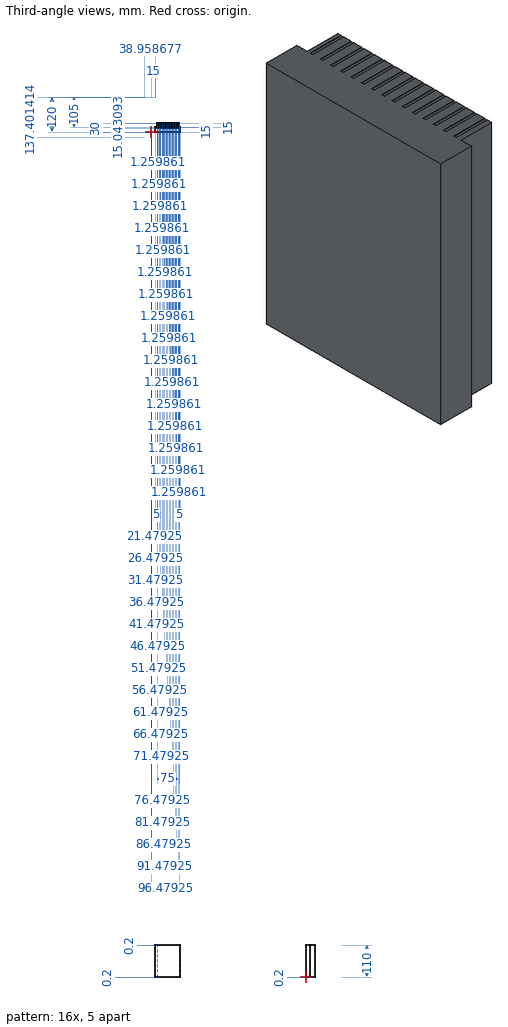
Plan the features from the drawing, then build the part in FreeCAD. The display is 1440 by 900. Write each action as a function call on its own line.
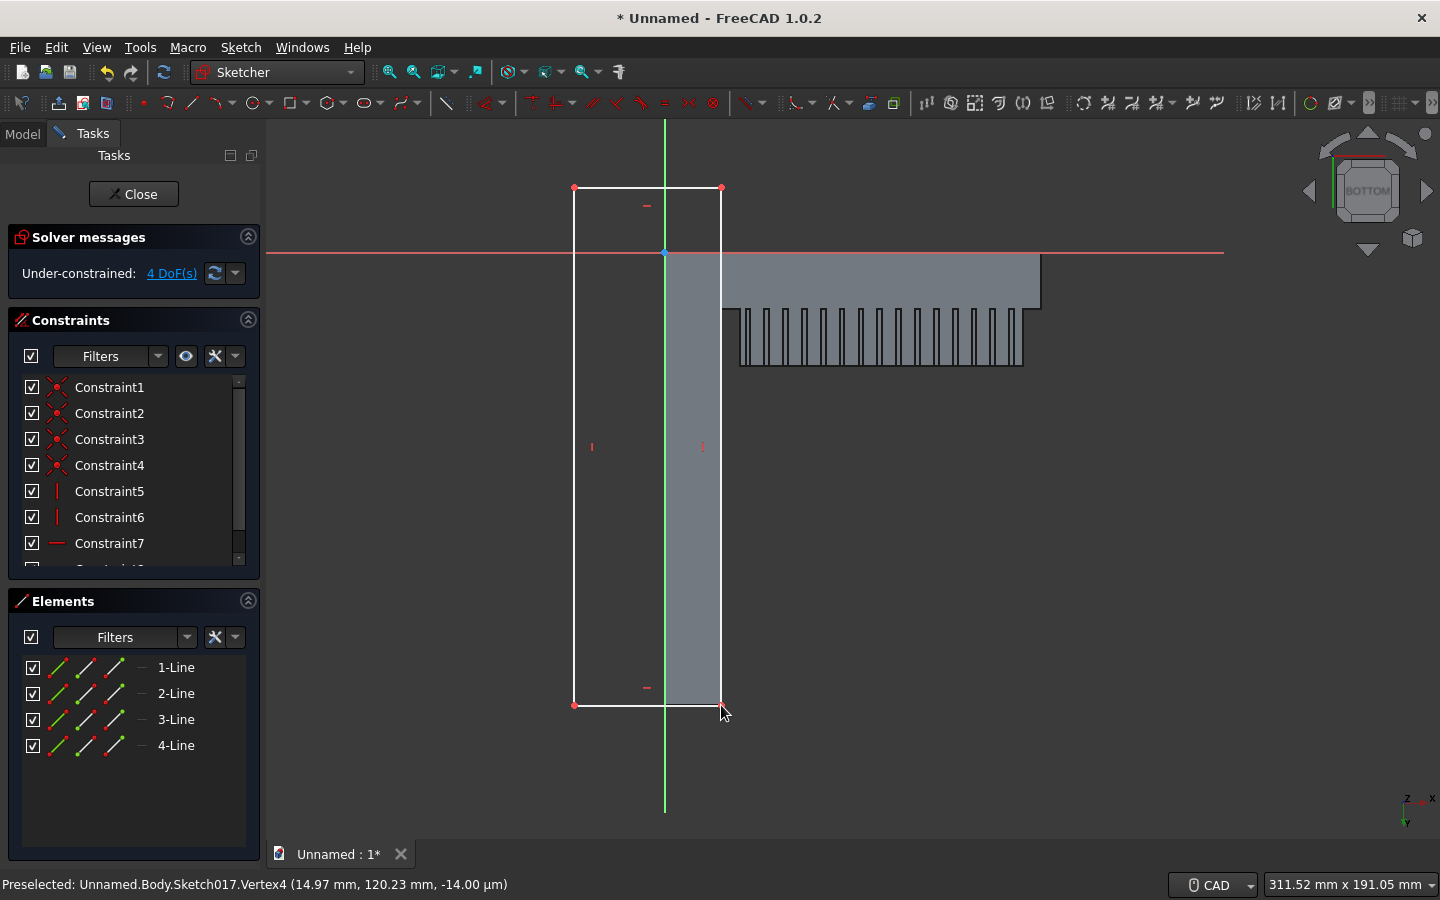
key(d)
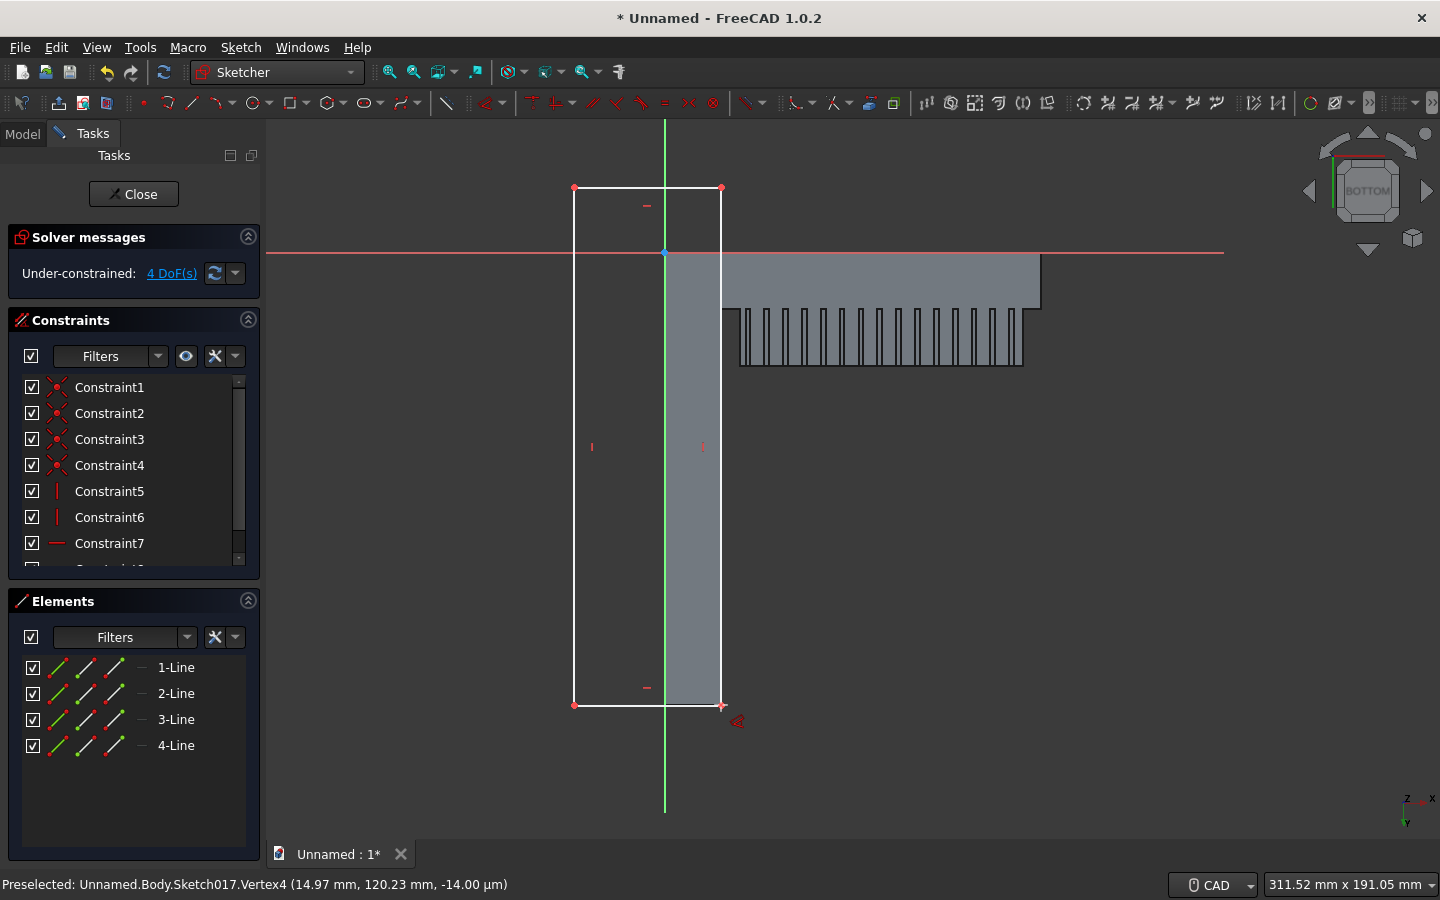
click(721, 706)
click(693, 740)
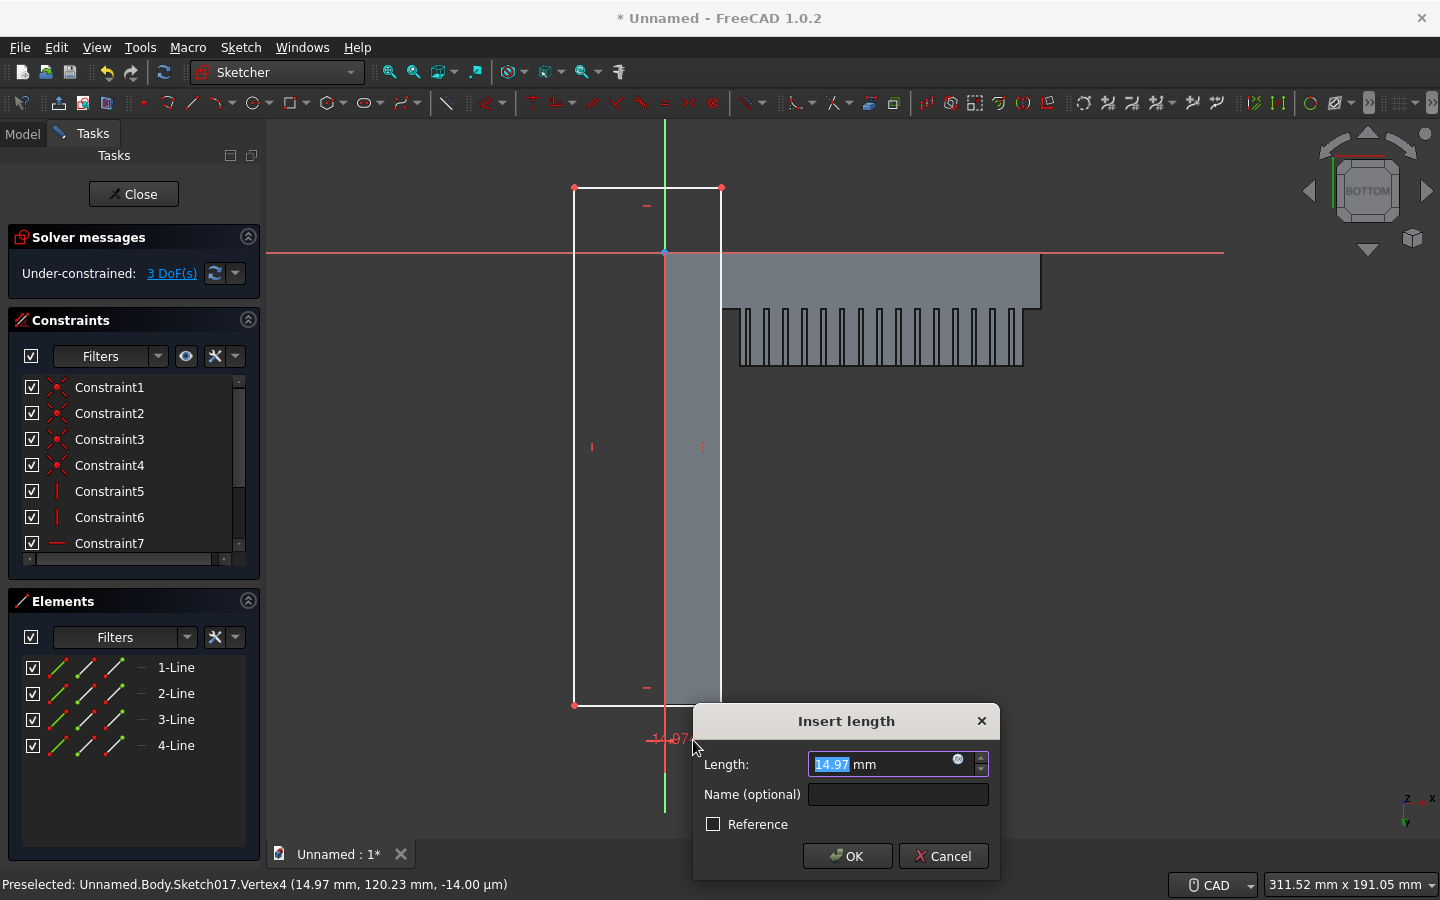
text(15)
key(Return)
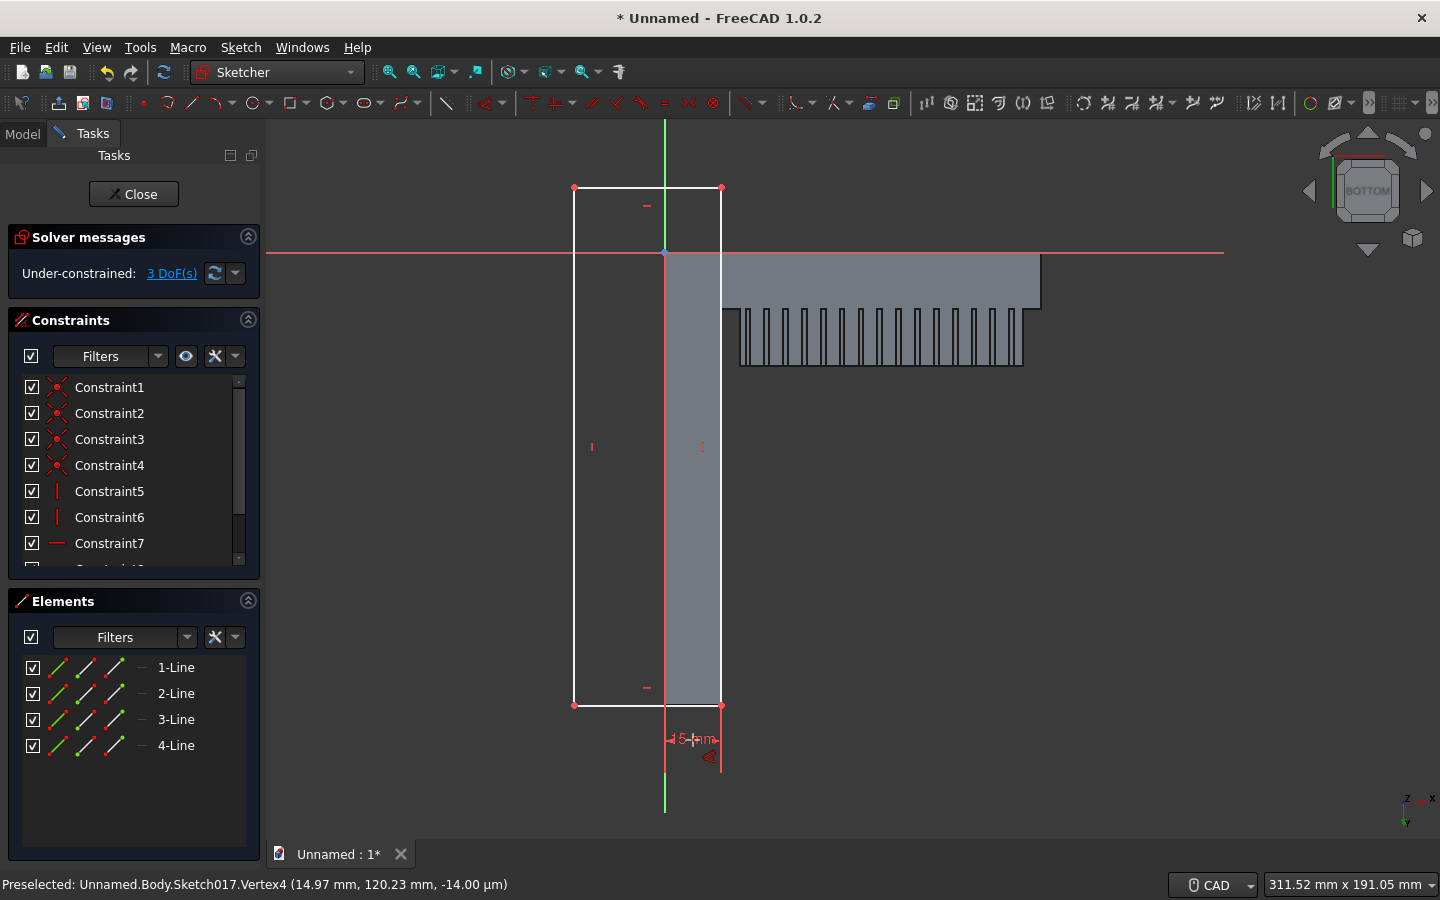
click(574, 706)
click(540, 479)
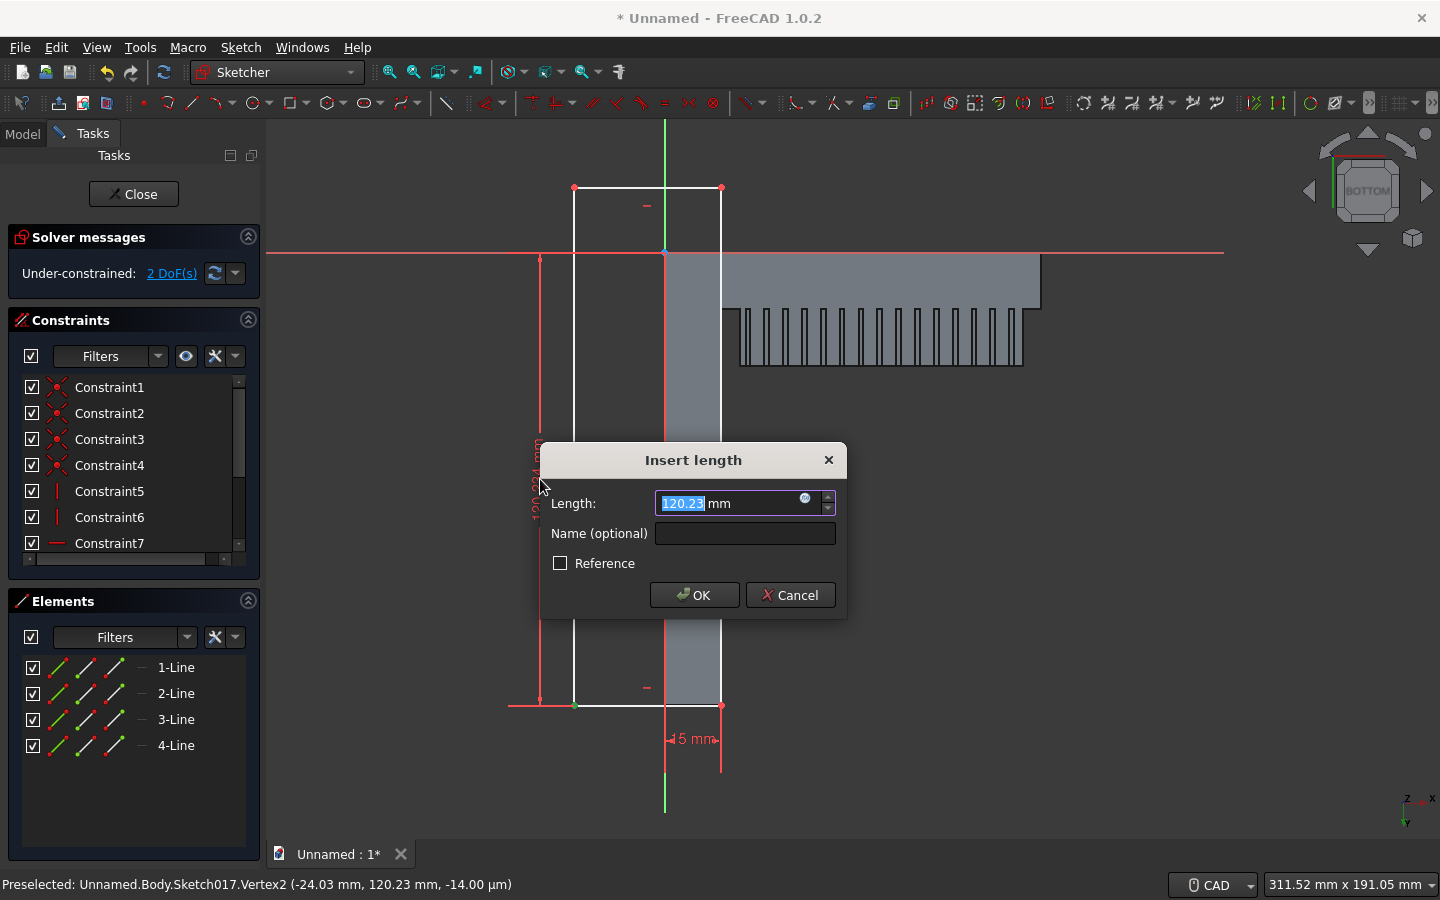
text(120)
key(Return)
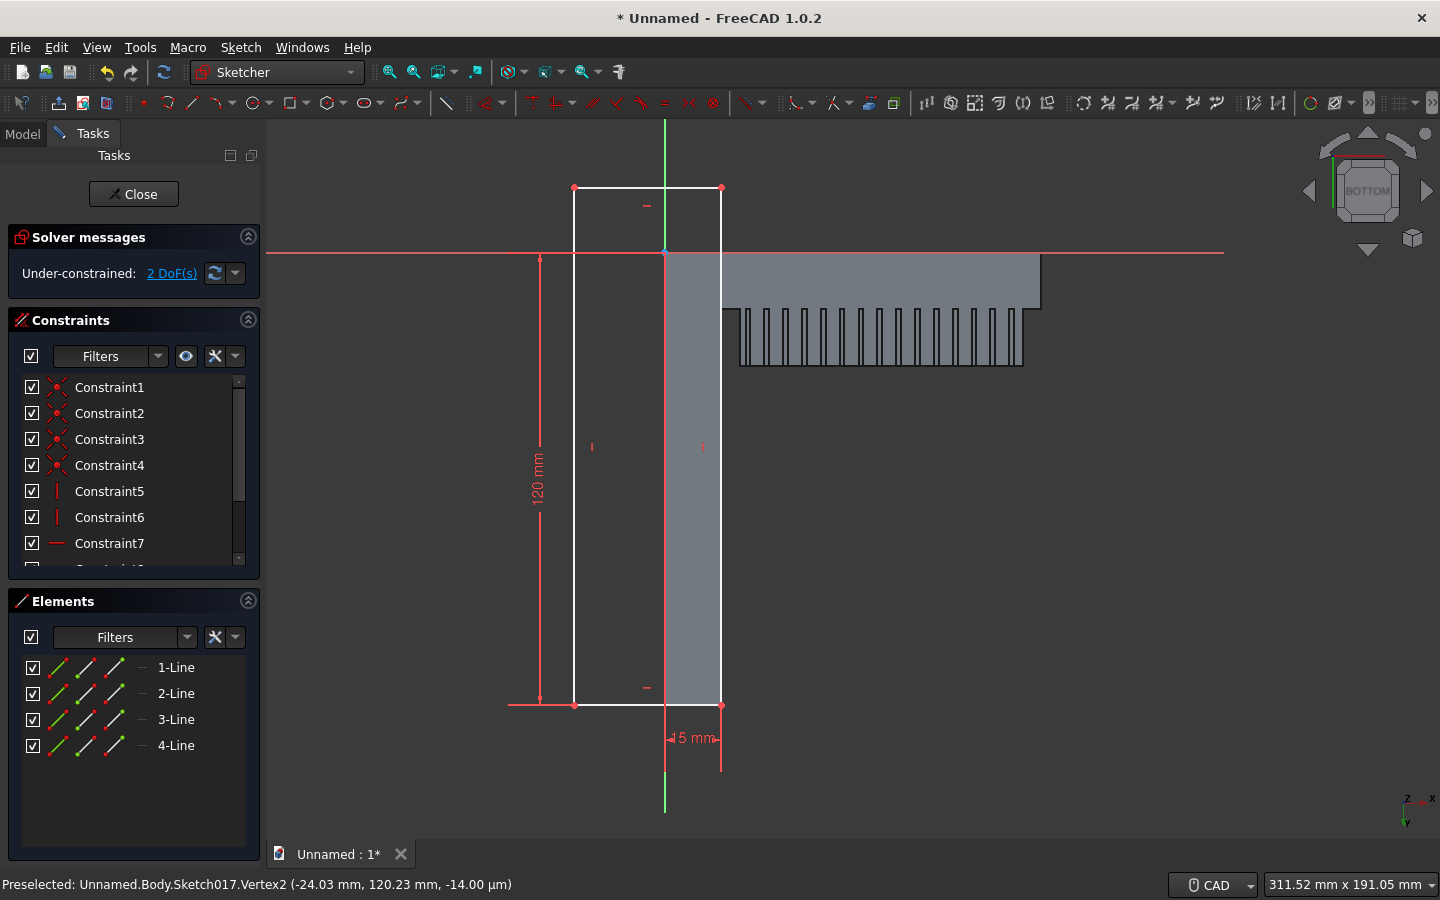
click(618, 705)
click(614, 739)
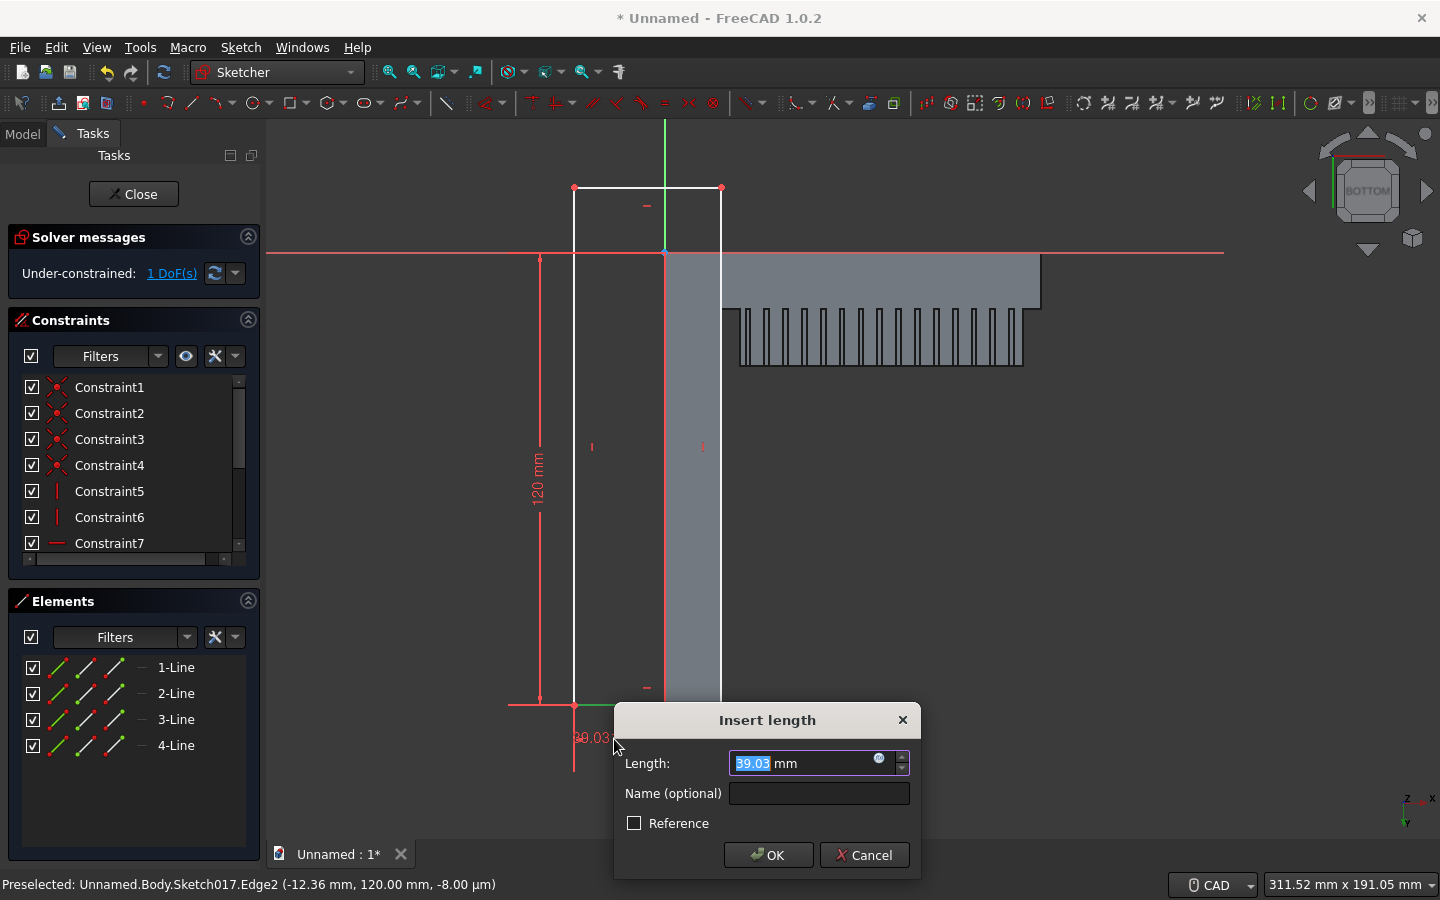
text(38.958677)
key(Return)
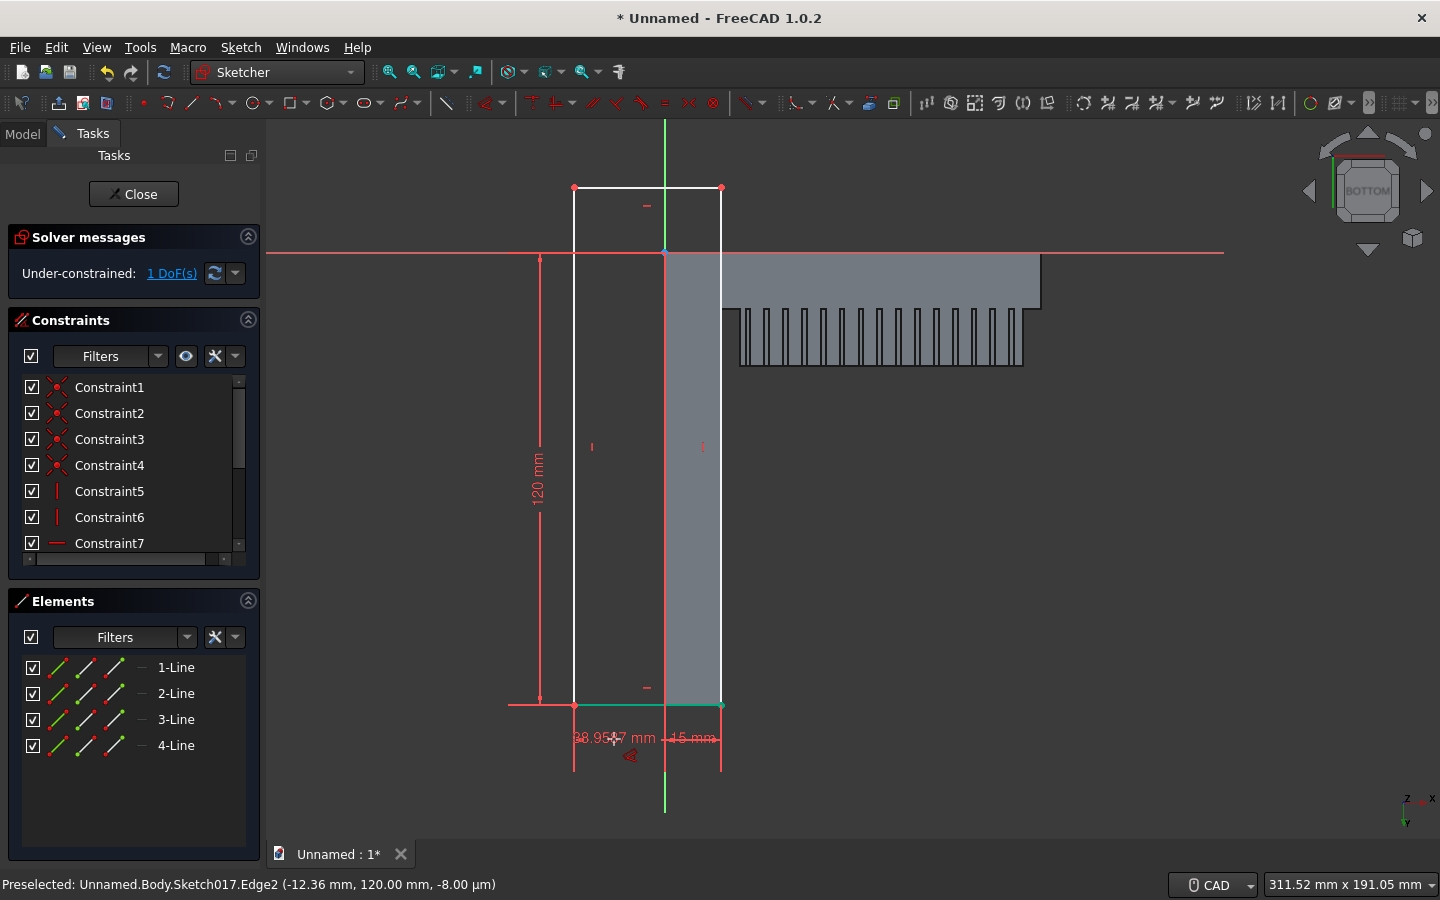
click(574, 343)
click(540, 447)